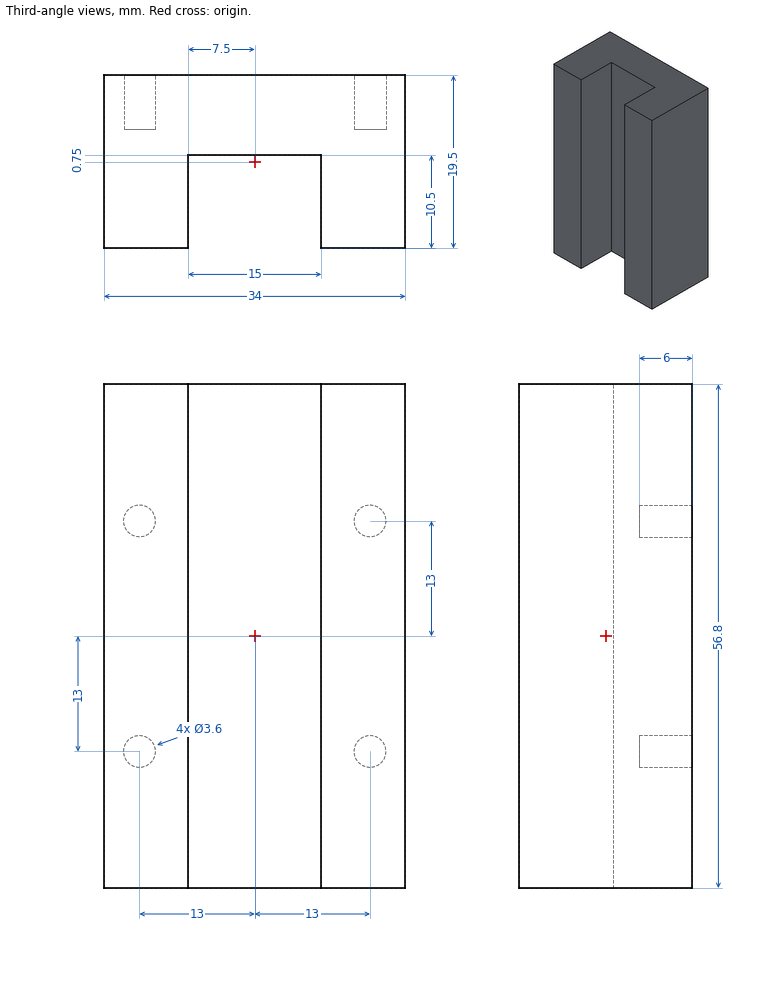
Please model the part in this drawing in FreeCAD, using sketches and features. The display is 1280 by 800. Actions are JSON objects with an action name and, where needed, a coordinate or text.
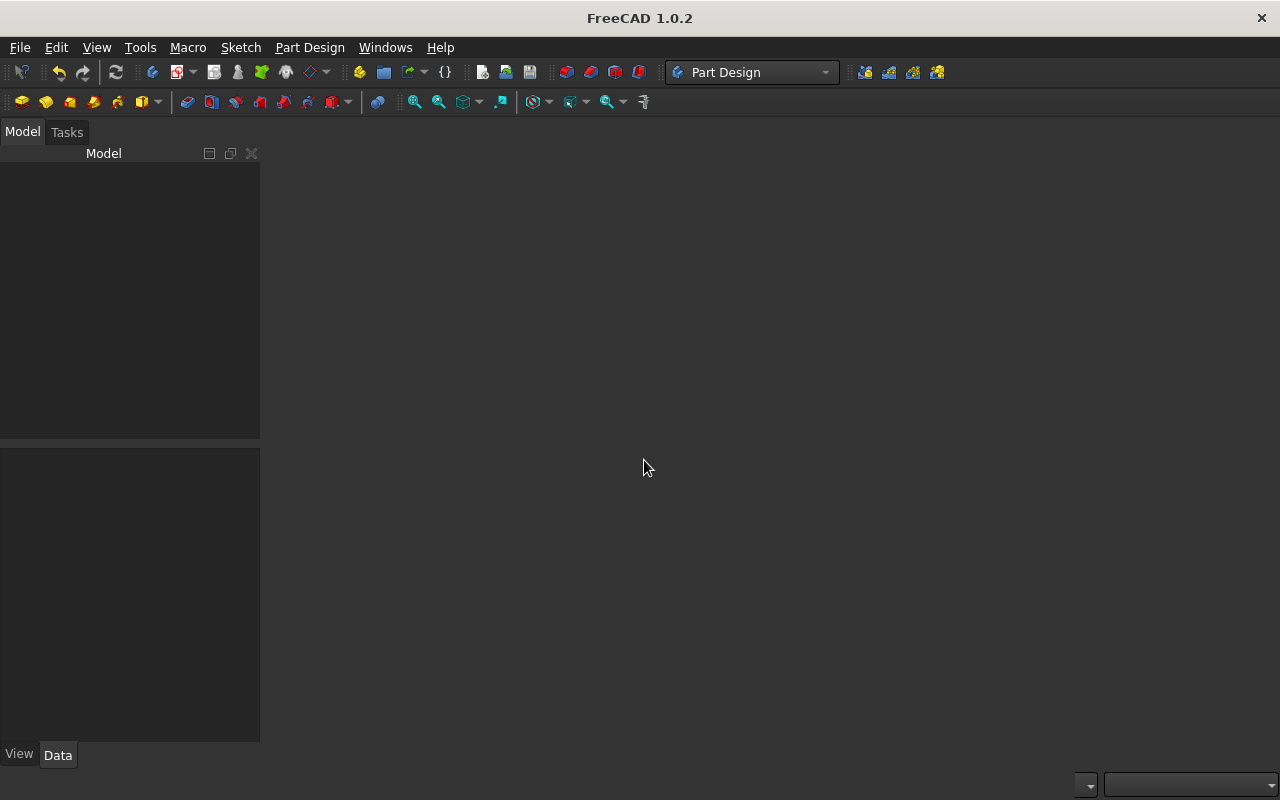
{"action": "left_click", "coordinate": [482, 72]}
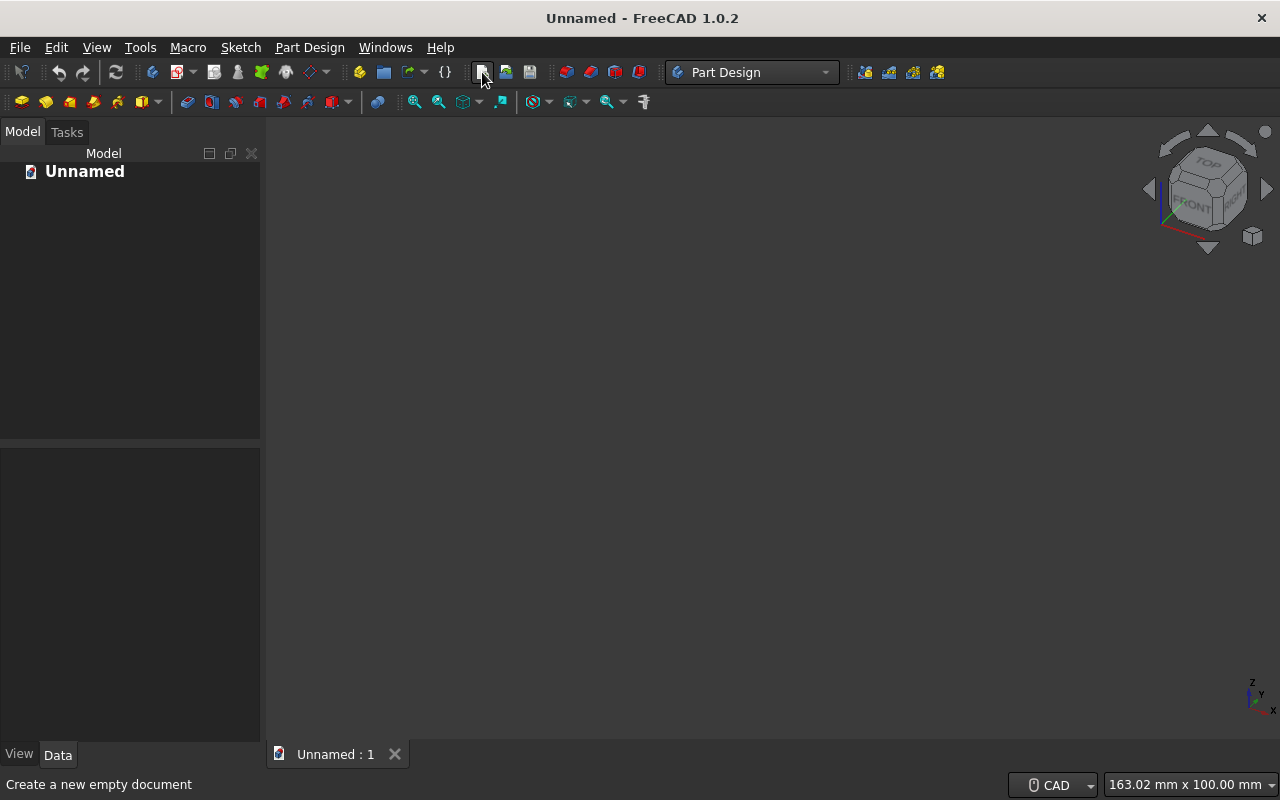
{"action": "left_click", "coordinate": [178, 72]}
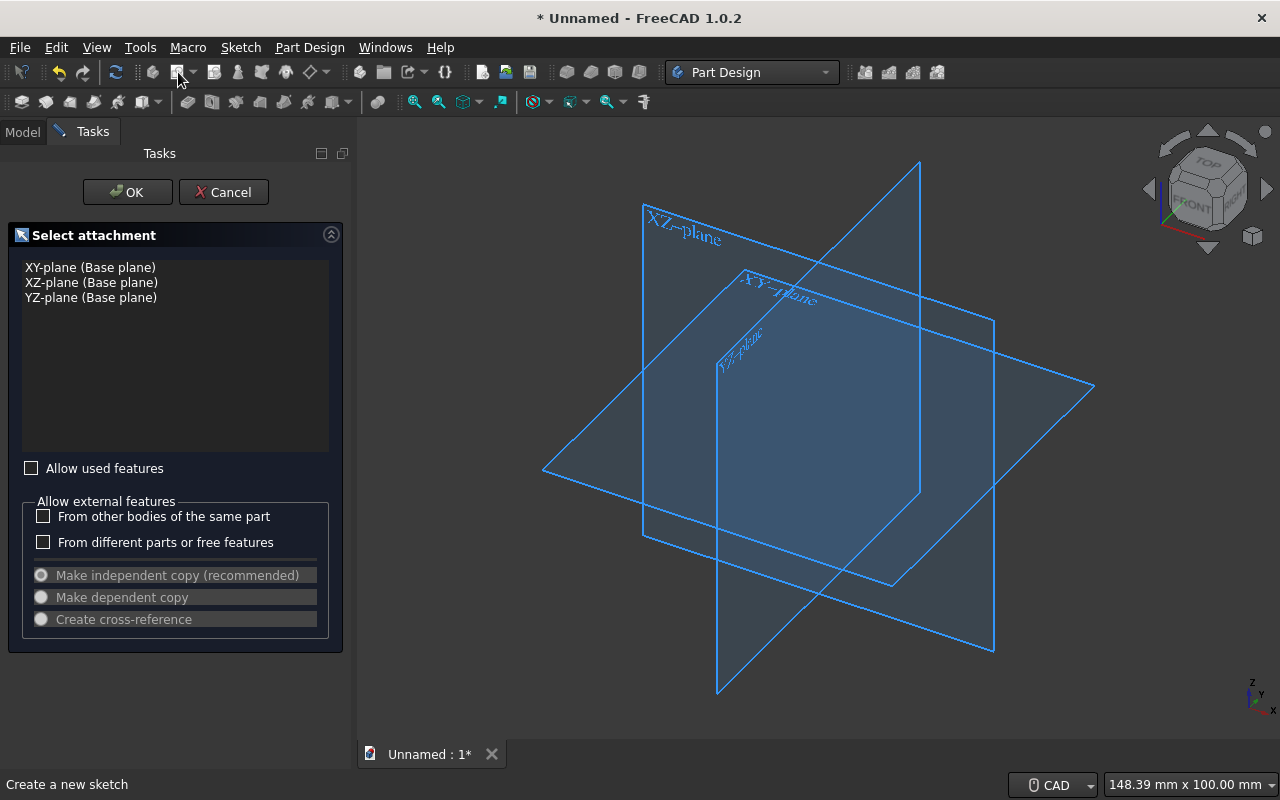
{"action": "left_click", "coordinate": [82, 268]}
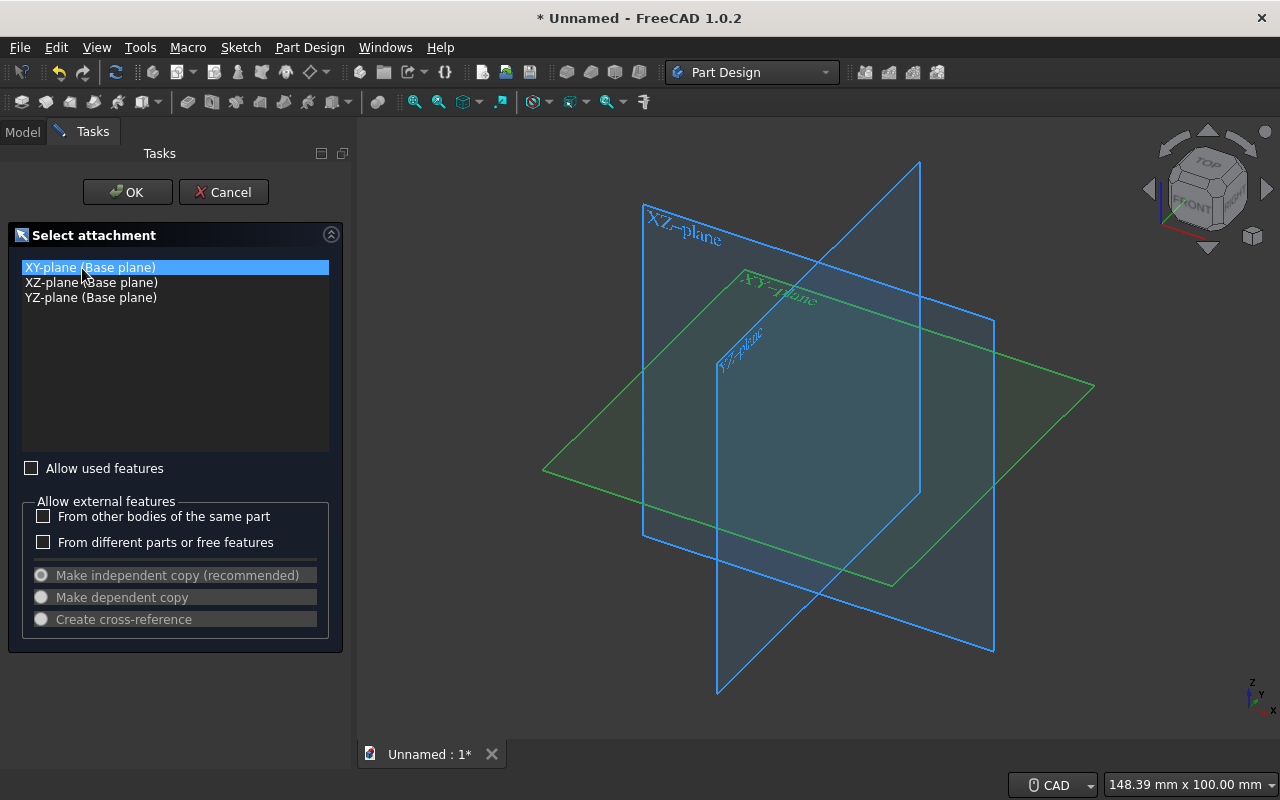
{"action": "left_click", "coordinate": [128, 192]}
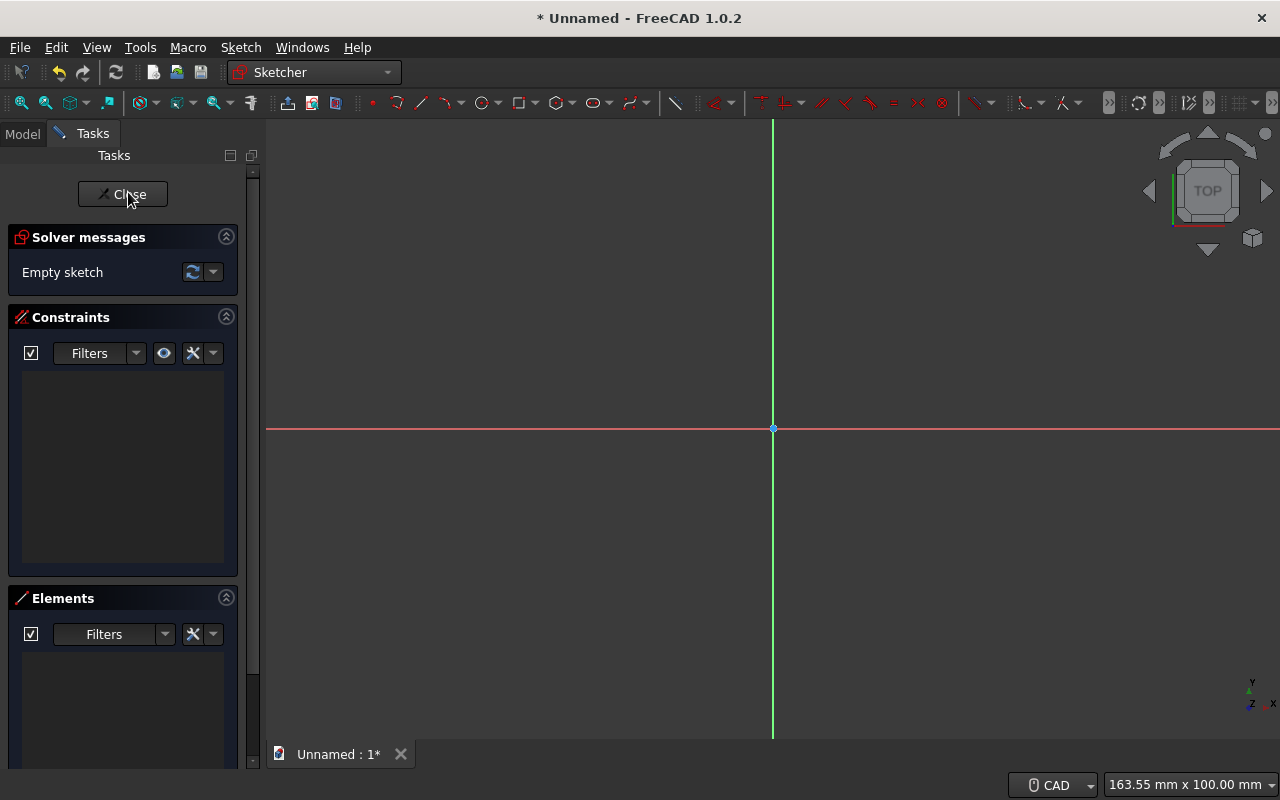
{"action": "scroll", "coordinate": [813, 429], "scroll_direction": "up", "scroll_amount": 5}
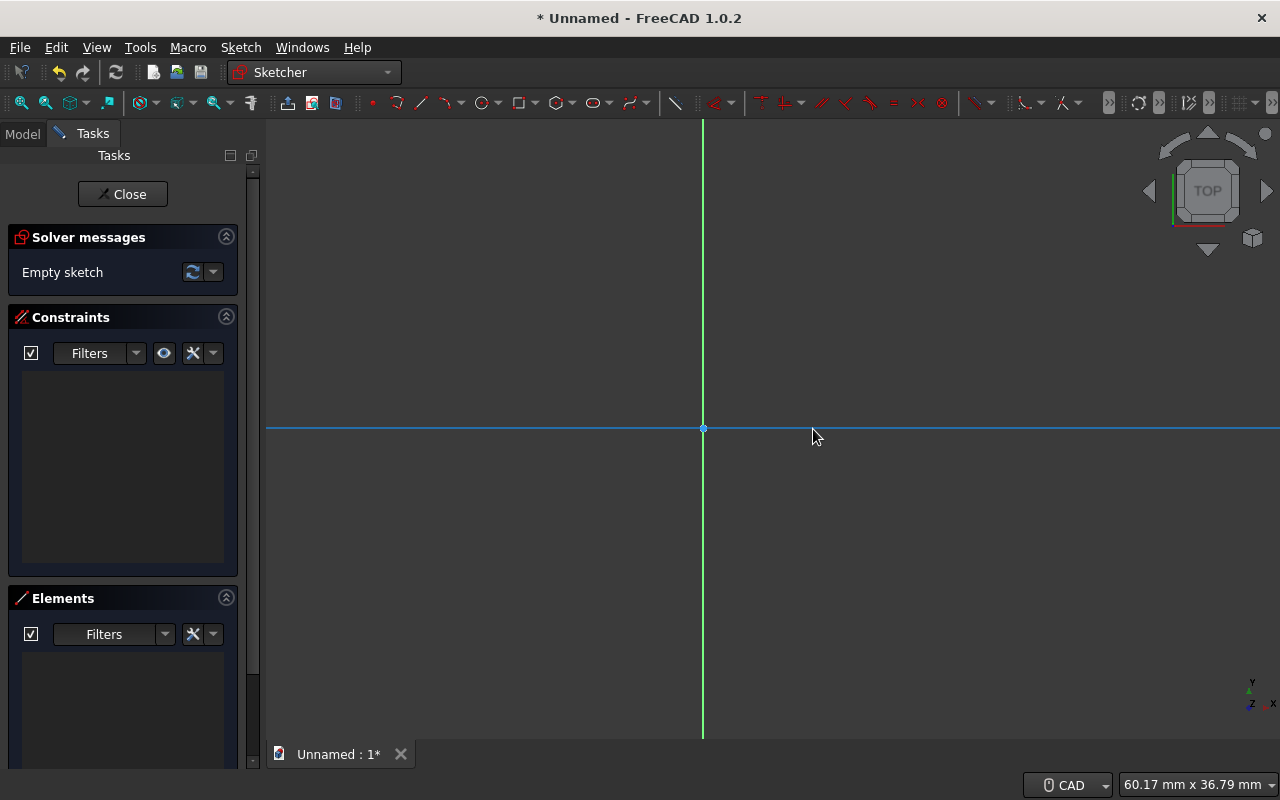
{"action": "key", "text": "g v"}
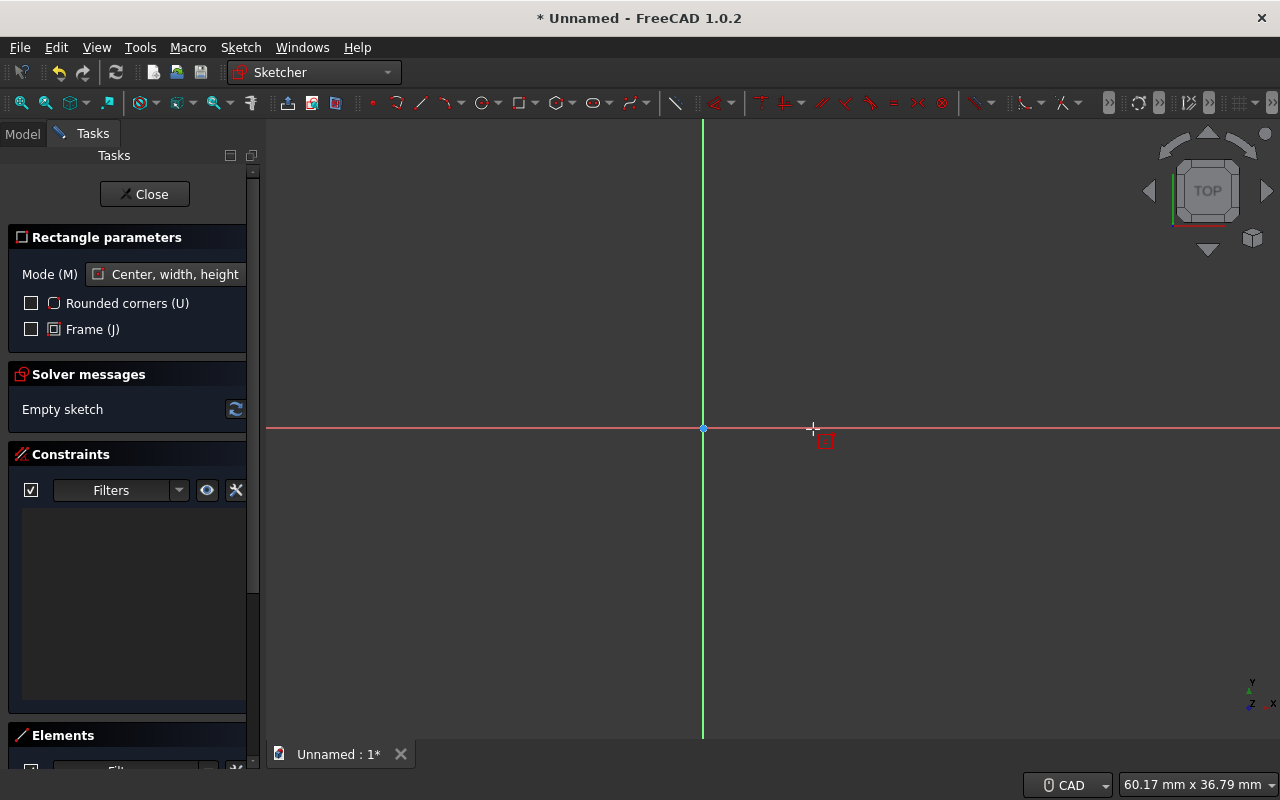
{"action": "left_click", "coordinate": [703, 428]}
{"action": "mouse_move", "coordinate": [990, 264]}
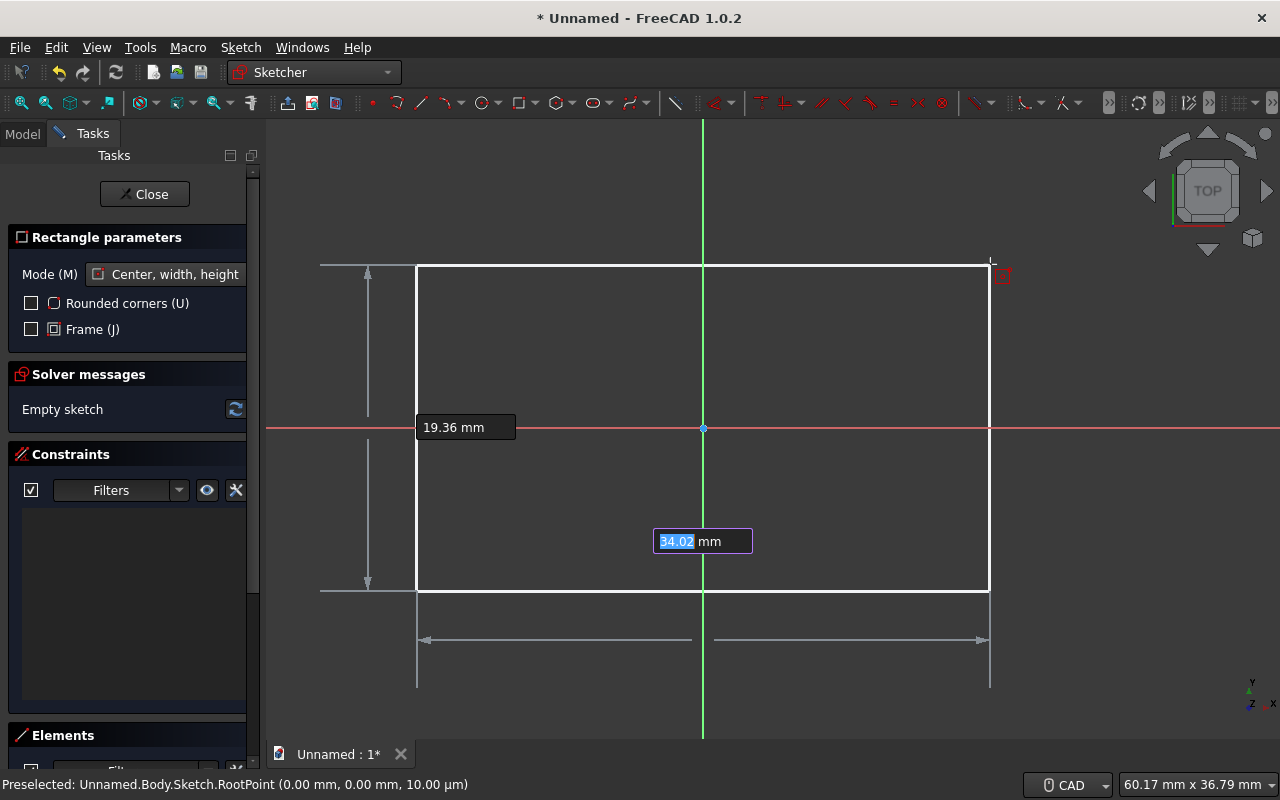
{"action": "type", "text": "34"}
{"action": "key", "text": "Tab"}
{"action": "type", "text": "19.5"}
{"action": "key", "text": "Return"}
{"action": "key", "text": "Escape"}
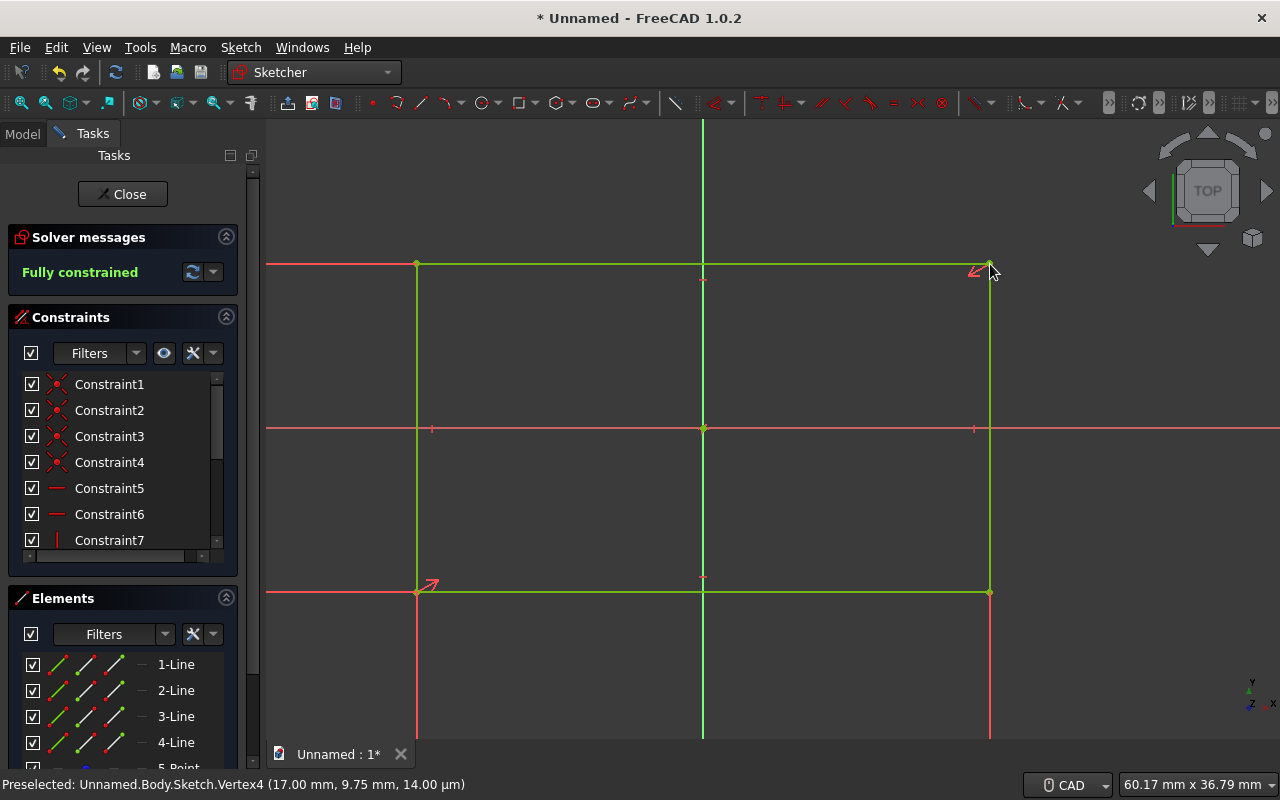
{"action": "left_click", "coordinate": [123, 194]}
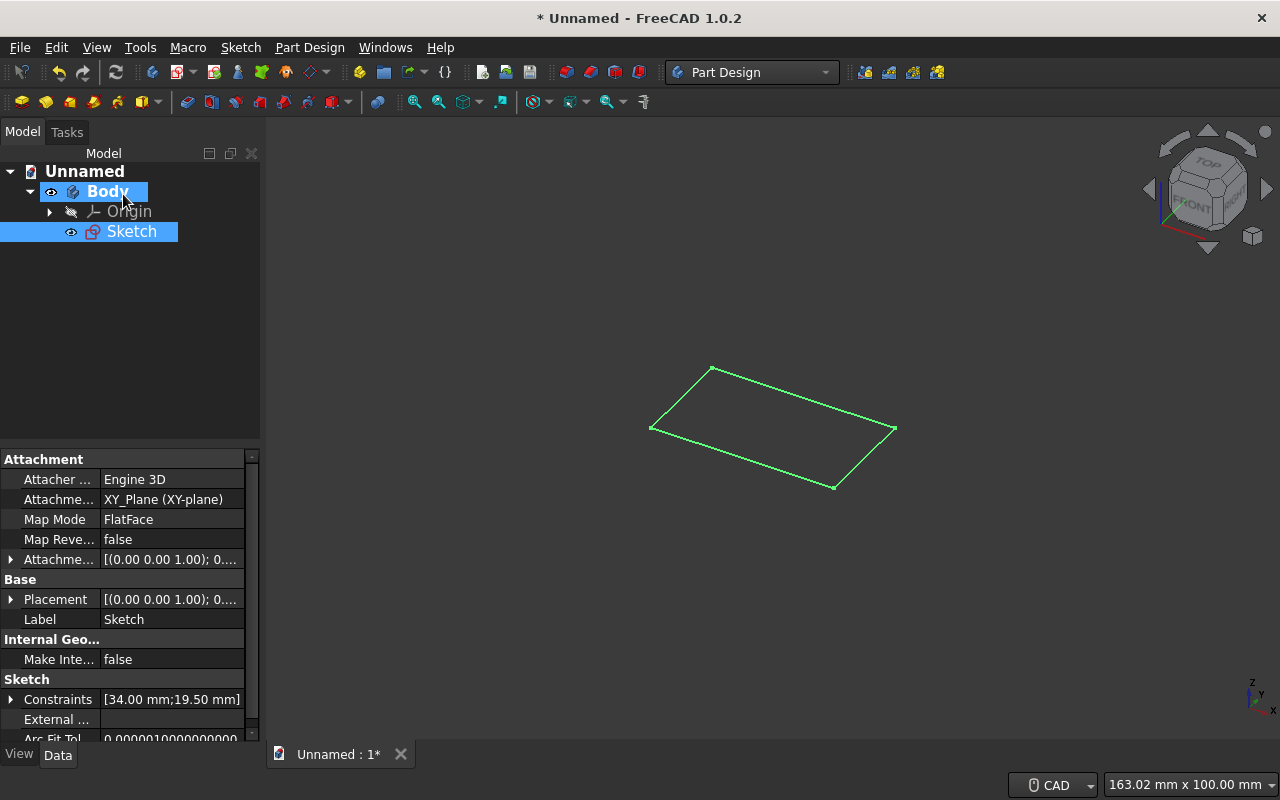
{"action": "left_click", "coordinate": [22, 102]}